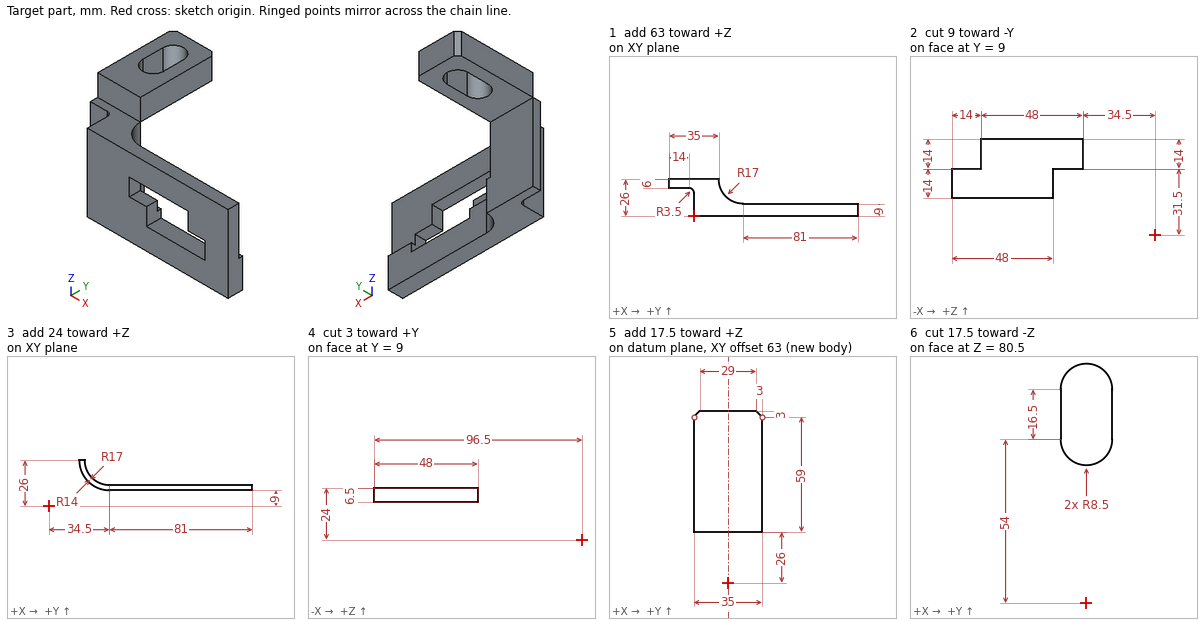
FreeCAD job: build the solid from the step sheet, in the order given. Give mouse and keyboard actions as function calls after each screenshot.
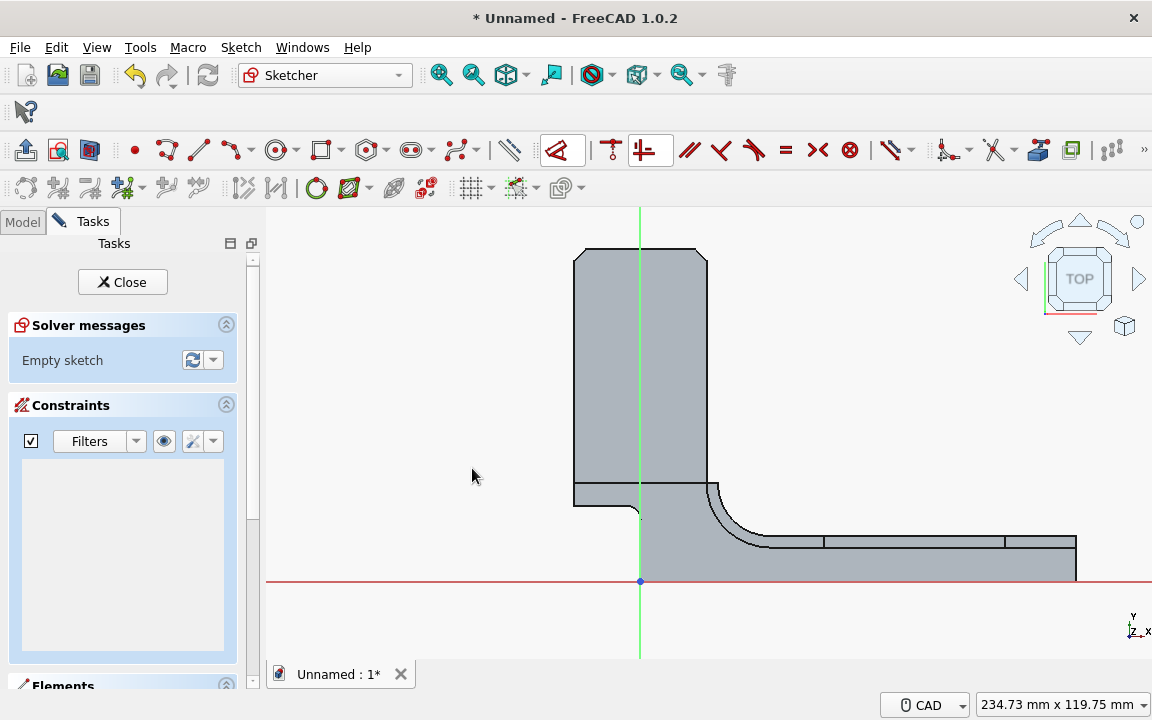
click(412, 150)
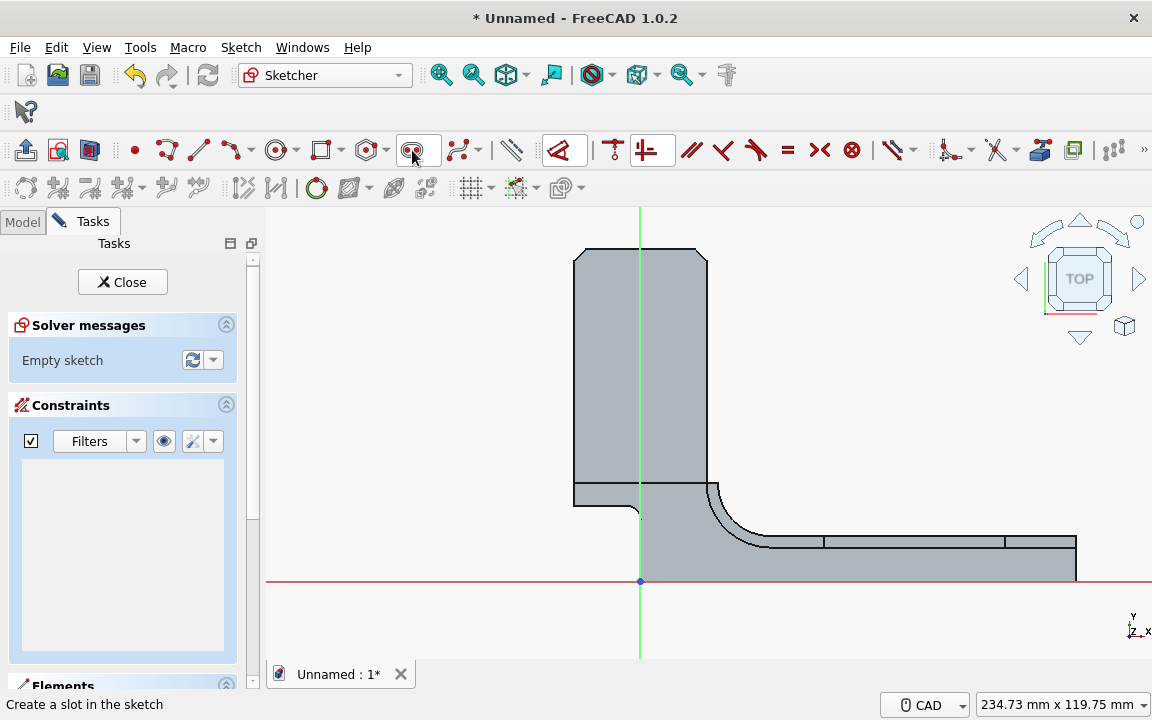
click(640, 378)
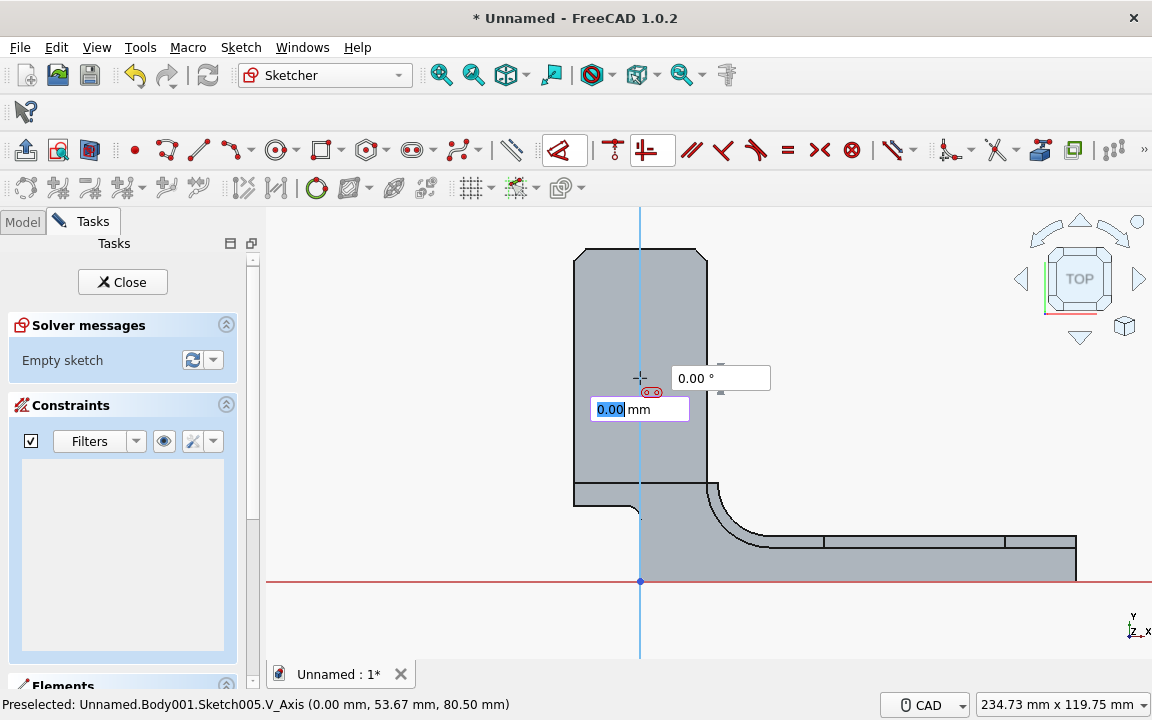
click(649, 315)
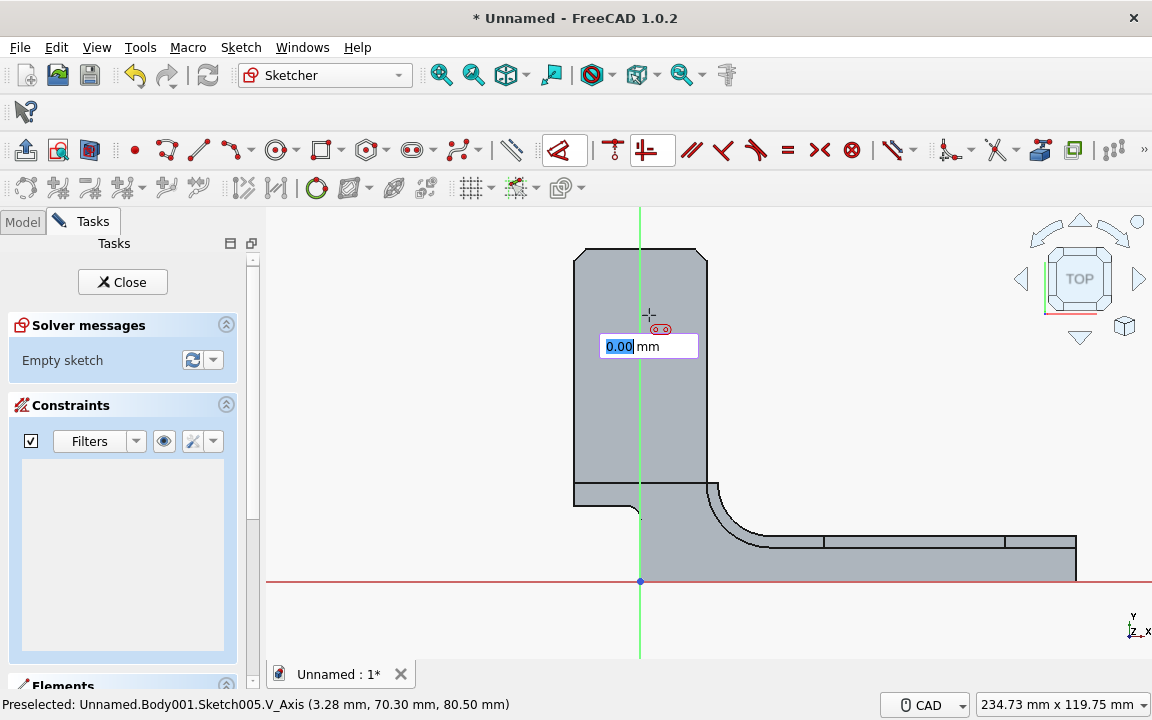
click(608, 347)
key(Escape)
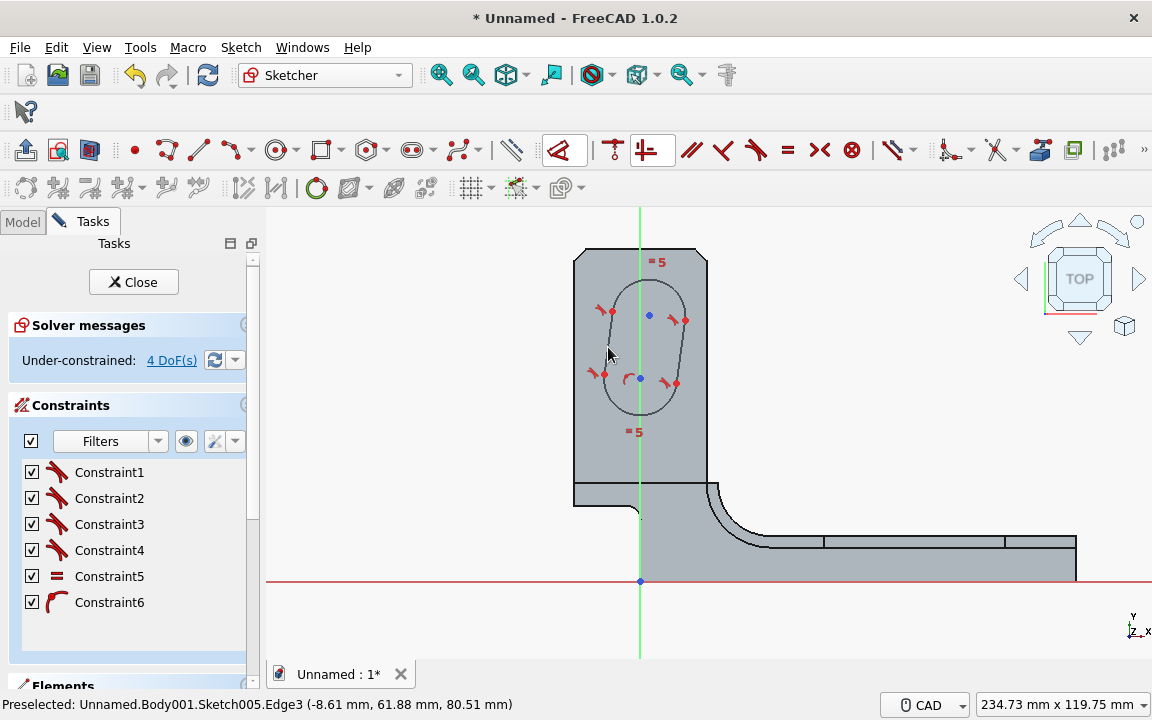
click(607, 355)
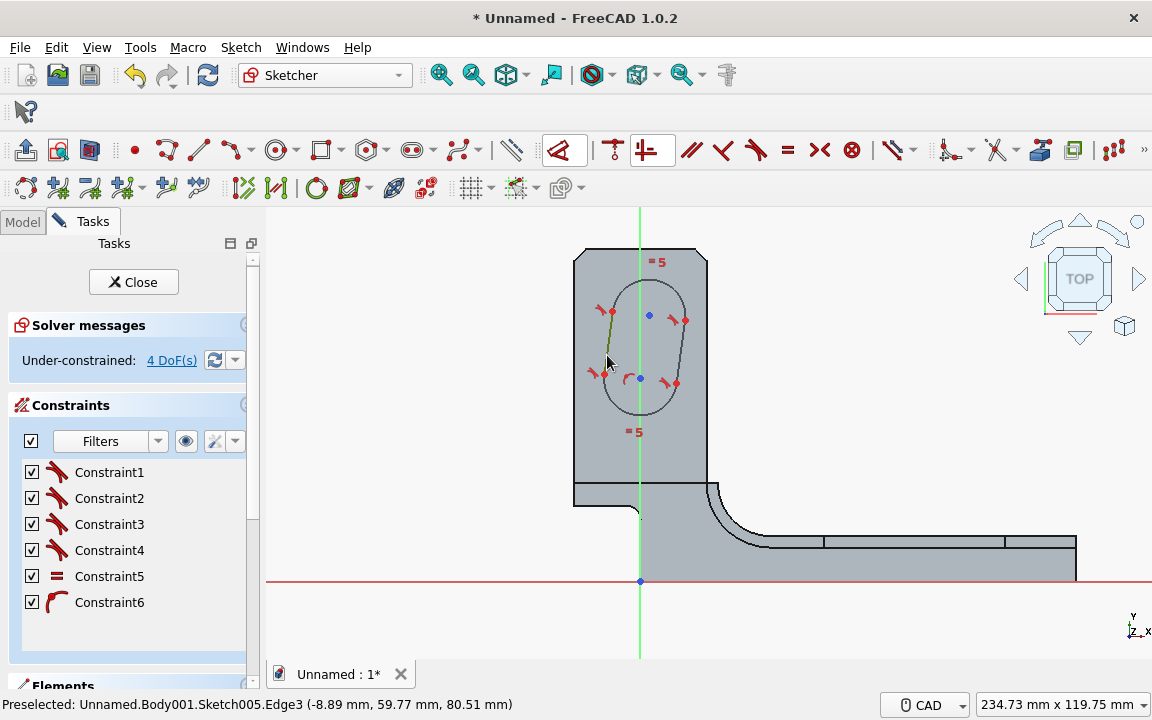
key(v)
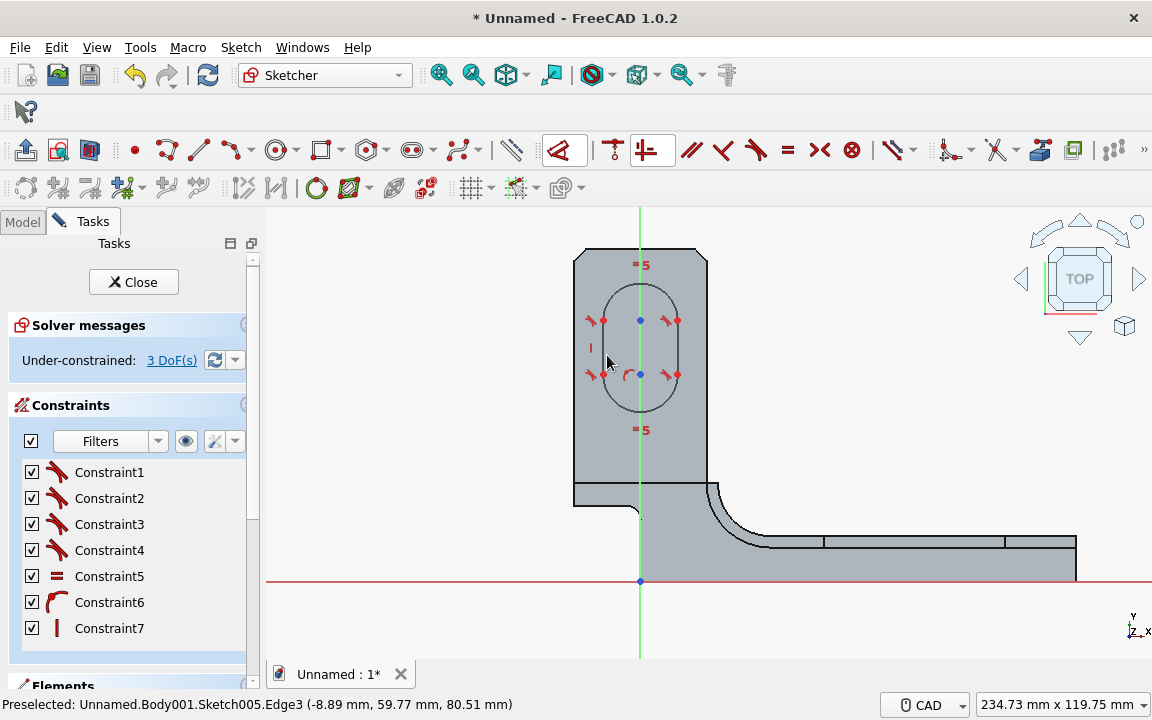
scroll(619, 405, up, 2)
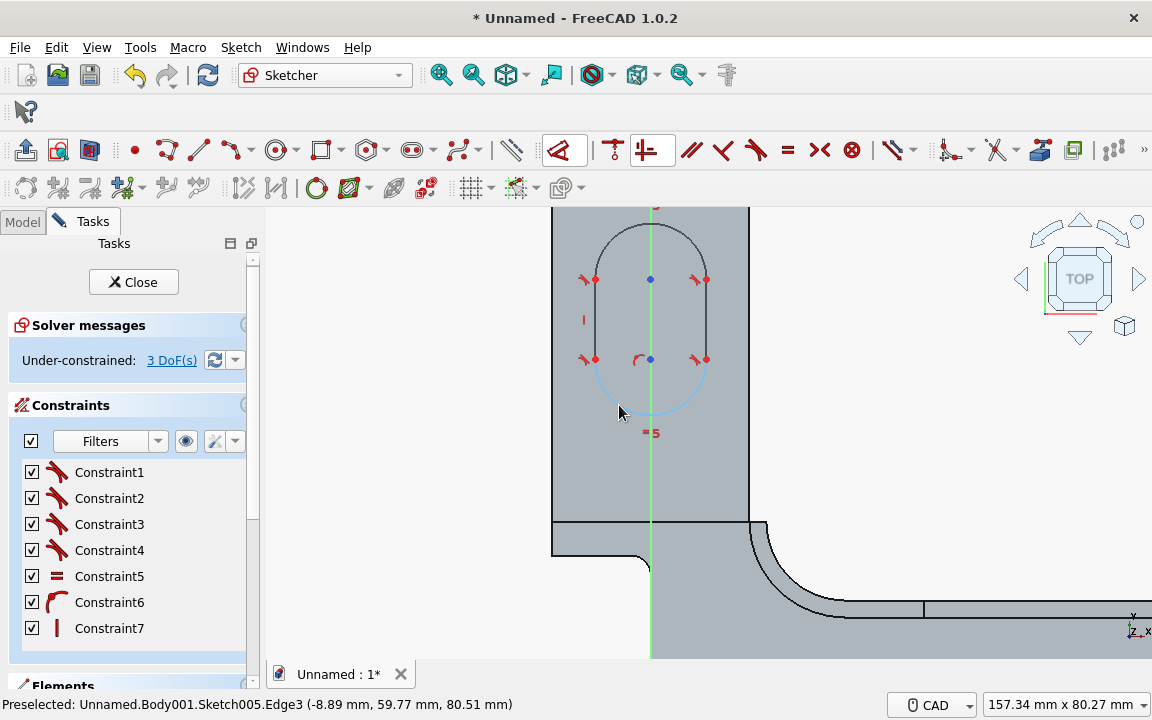
click(618, 405)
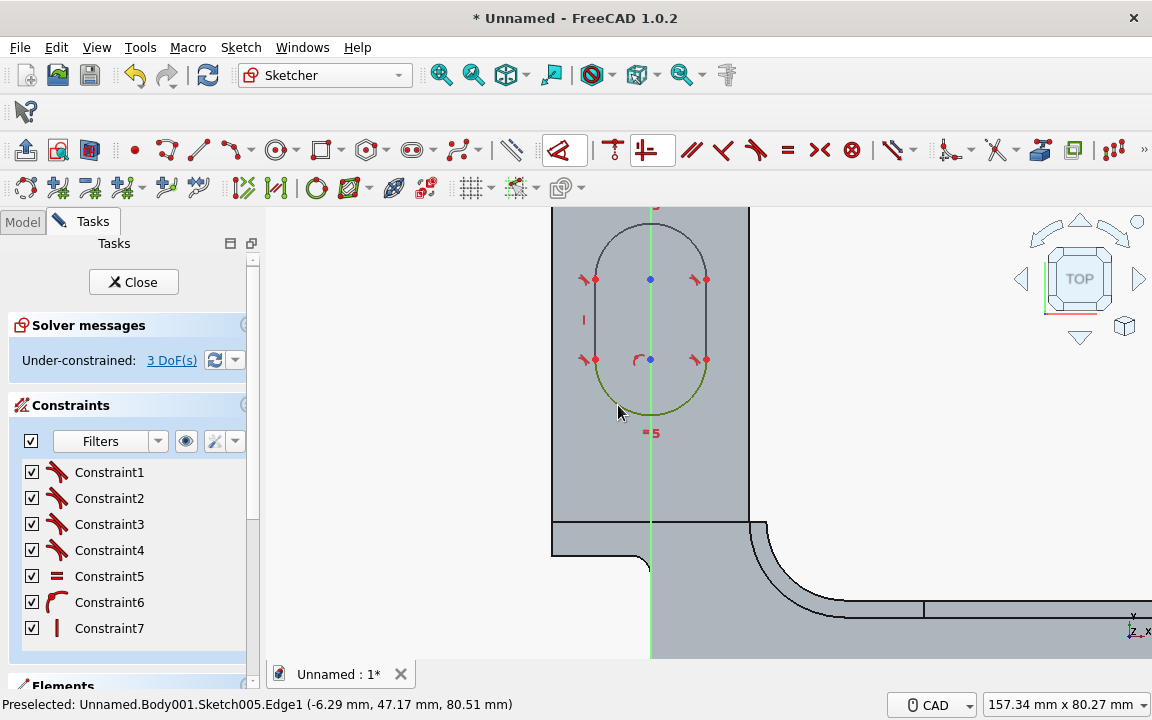
key(k)
key(r)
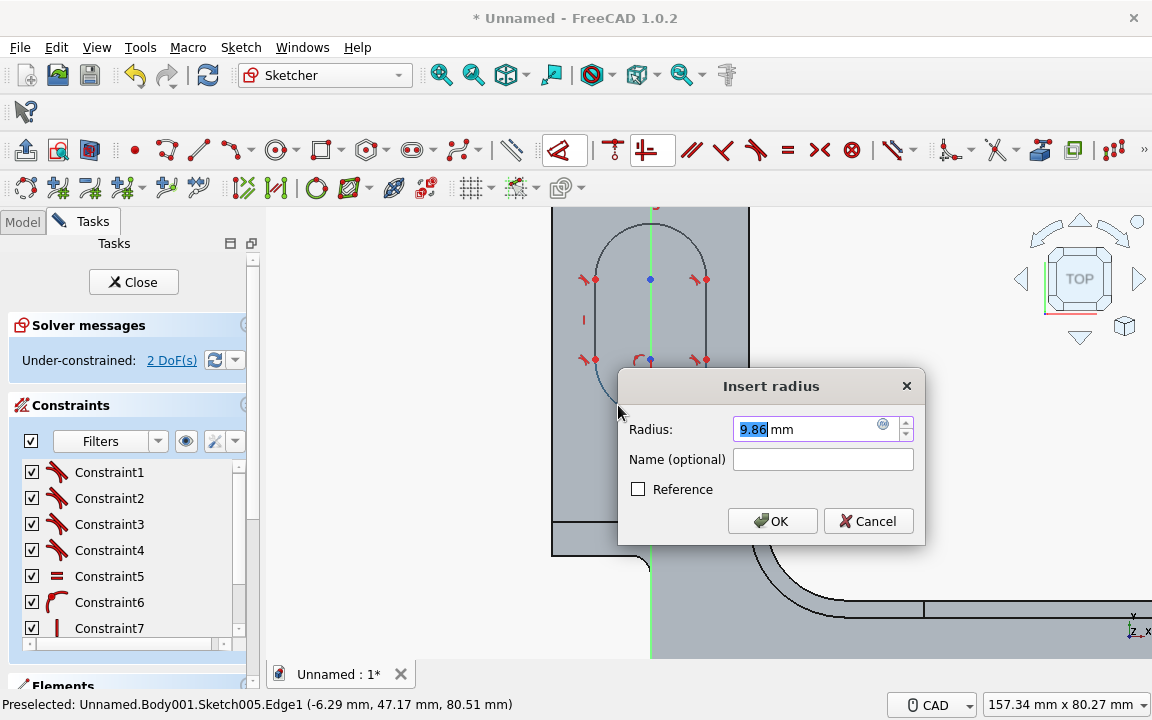
text(8.5)
key(Return)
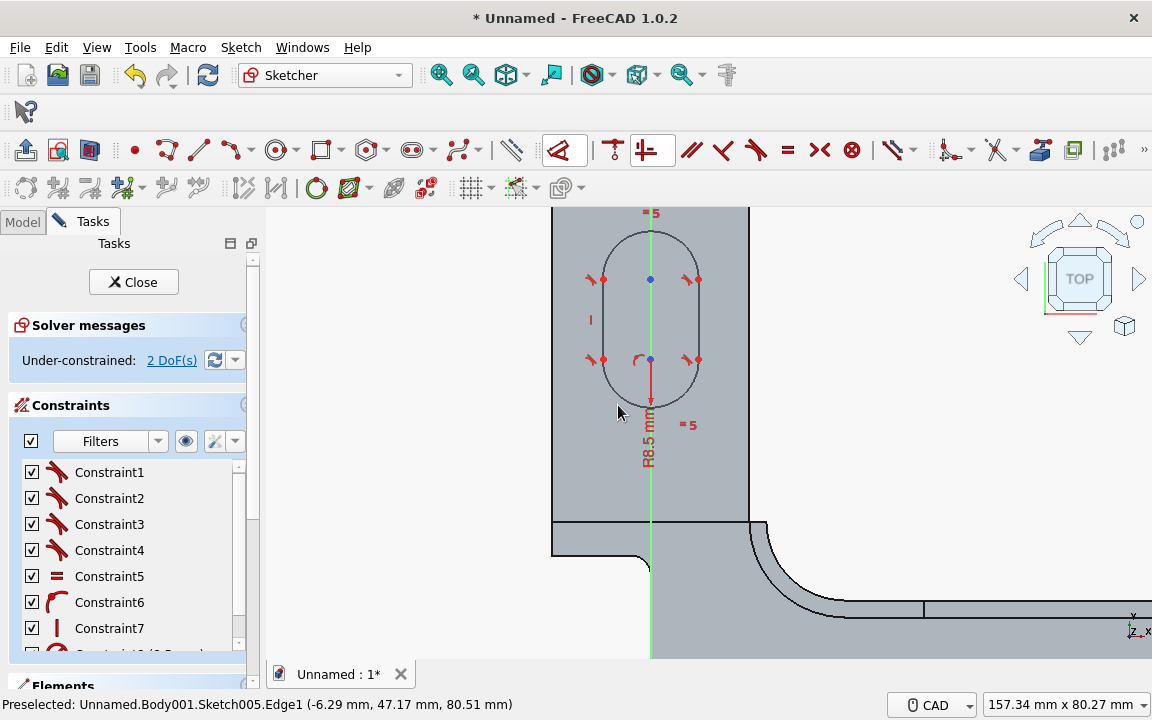
click(603, 360)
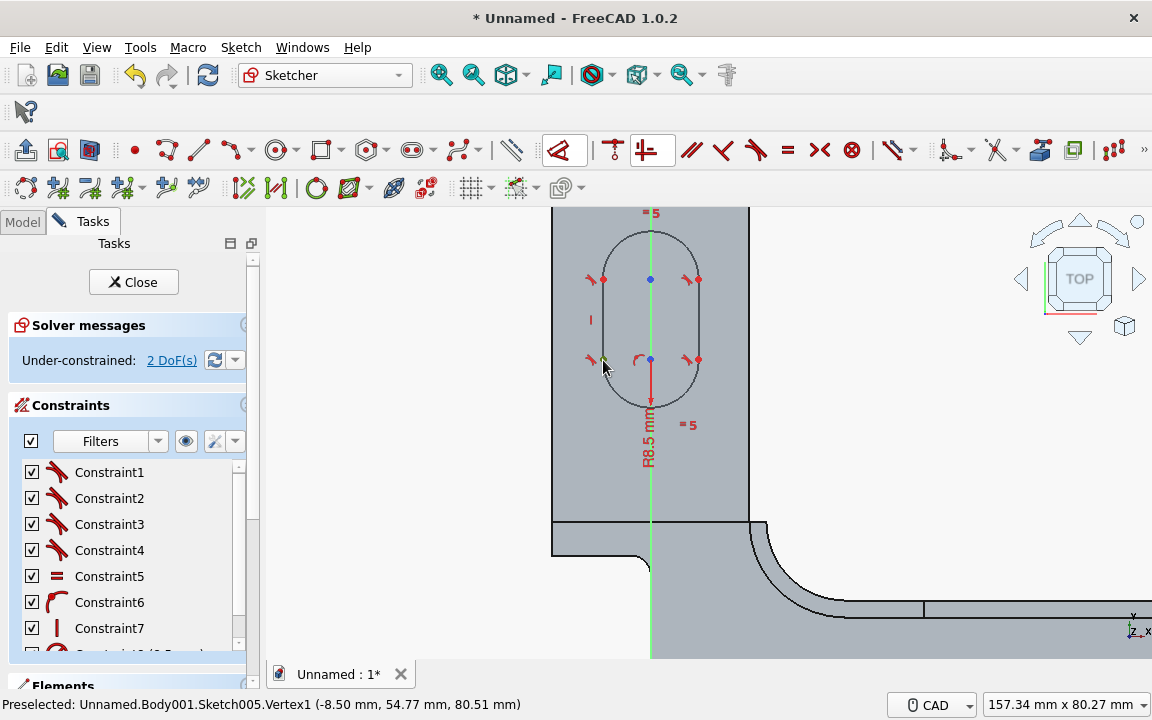
key(i)